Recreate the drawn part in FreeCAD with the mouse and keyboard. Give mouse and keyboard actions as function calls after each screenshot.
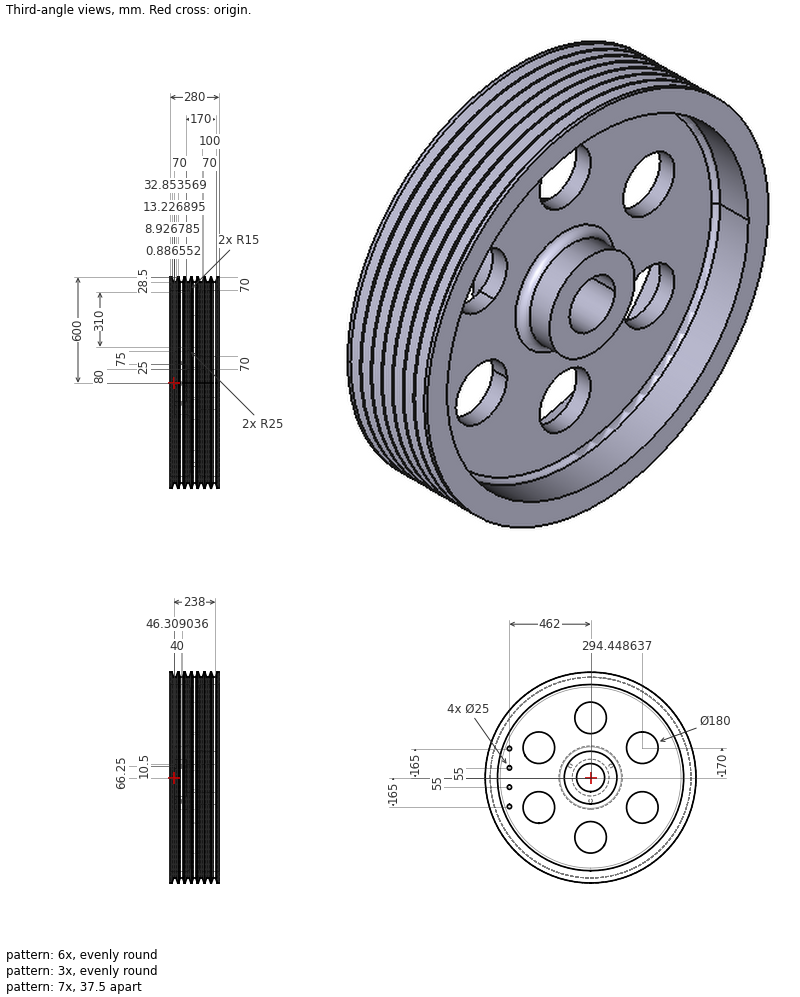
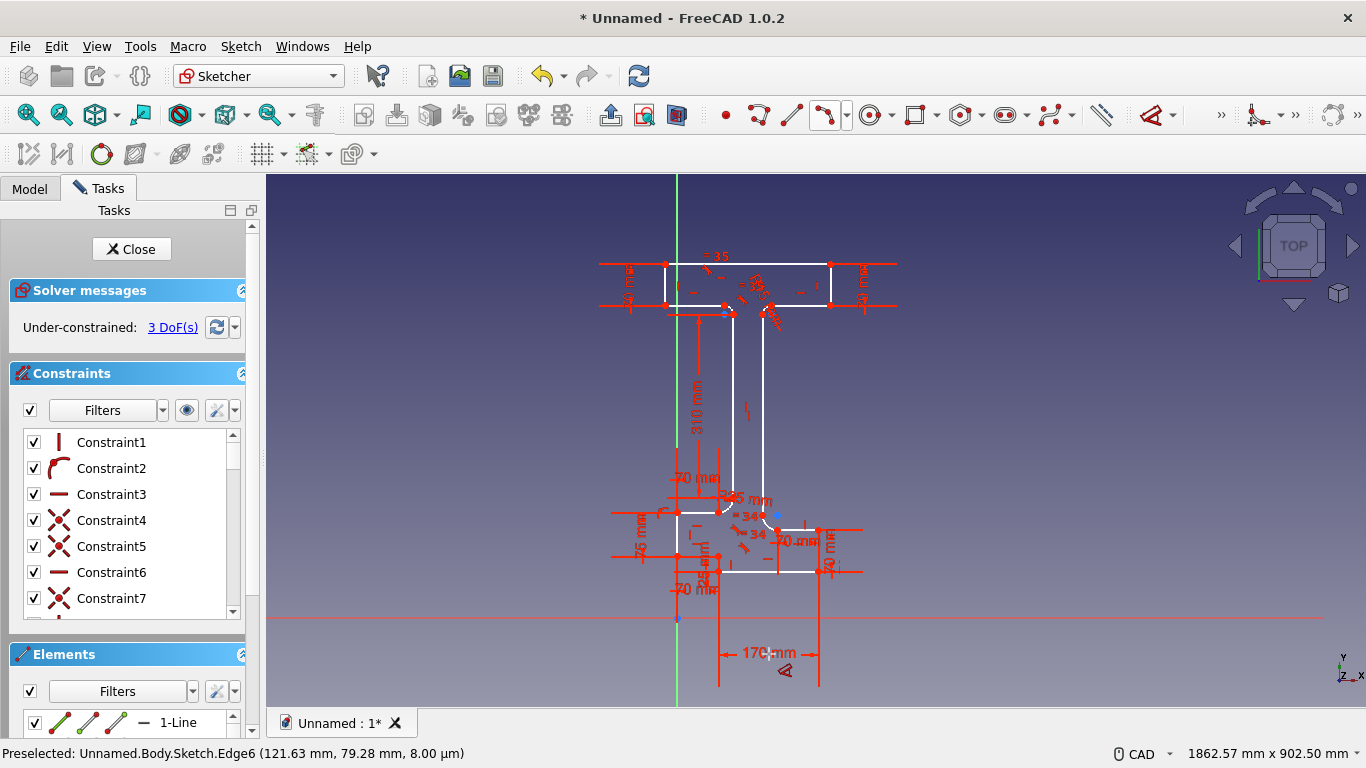
click(789, 306)
click(801, 340)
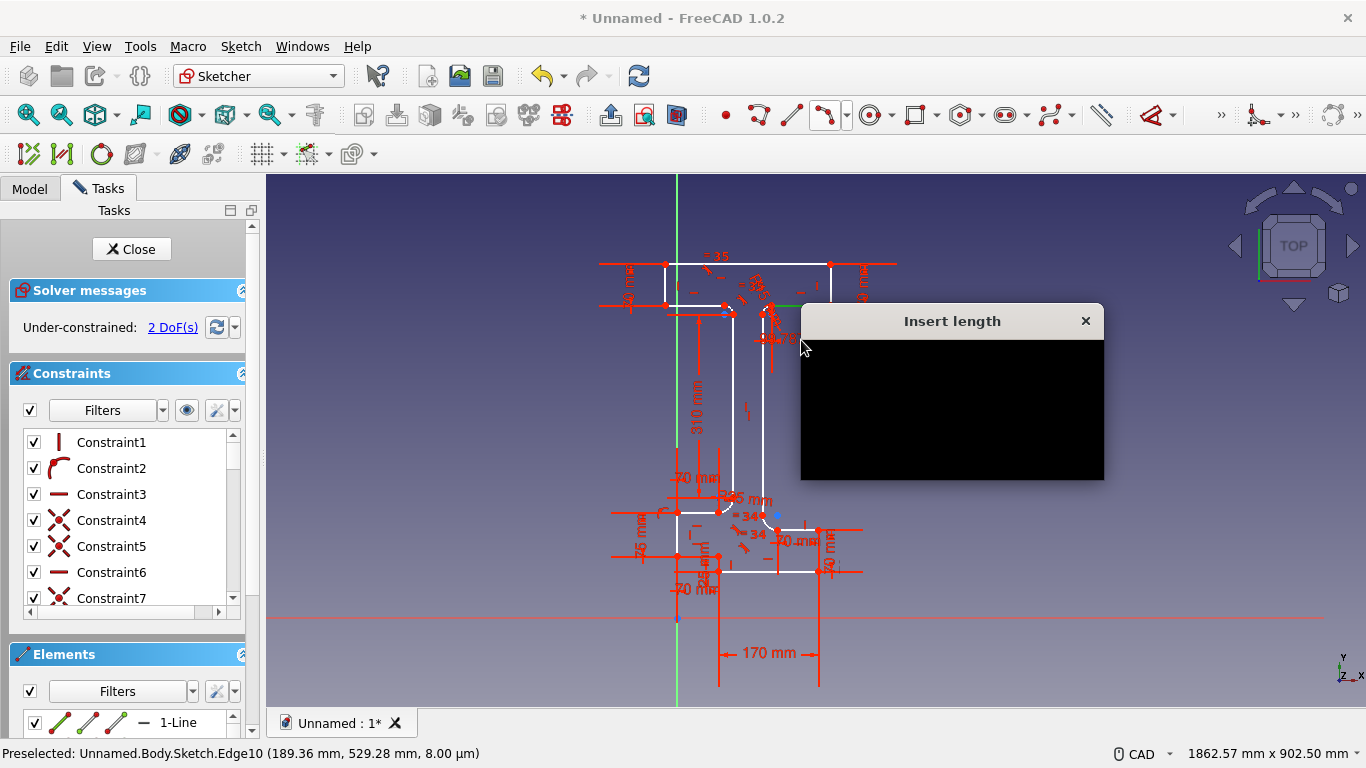
text(100)
key(Return)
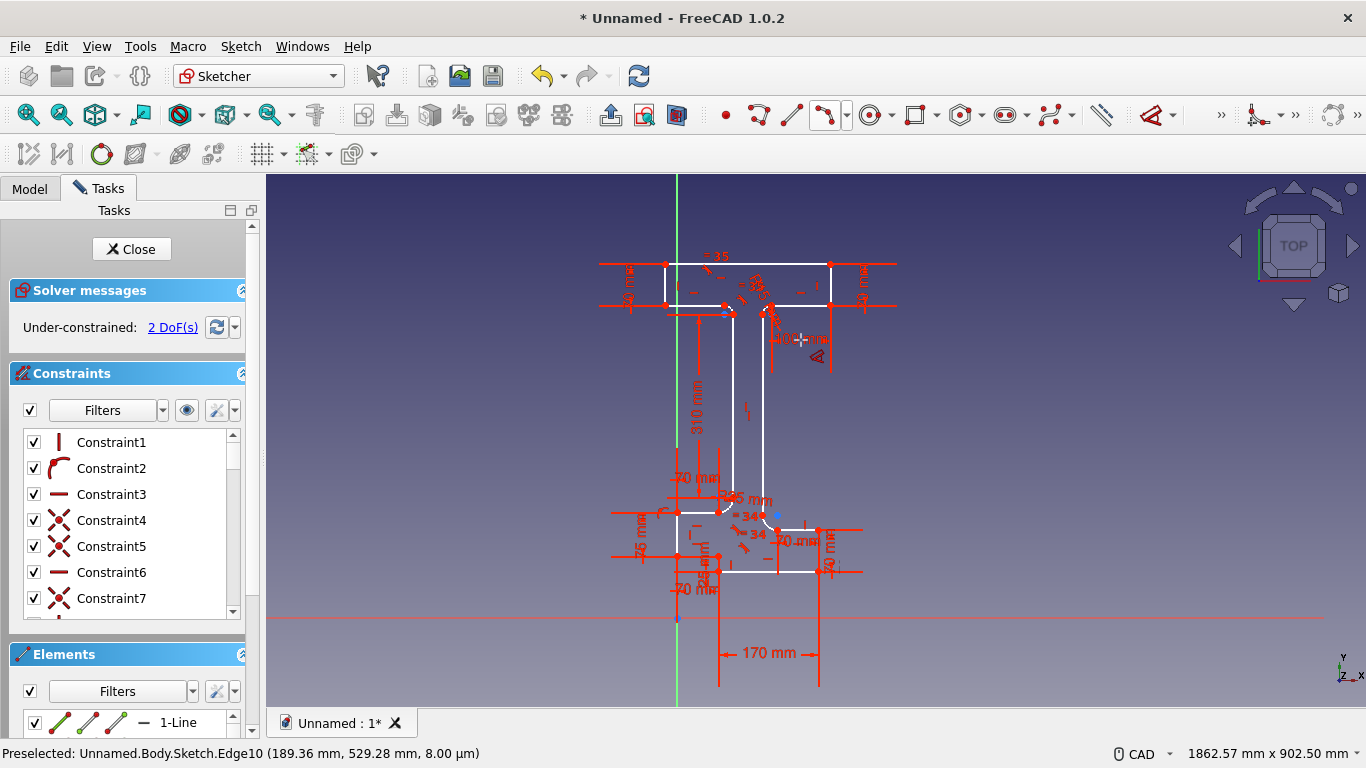
click(781, 264)
click(748, 230)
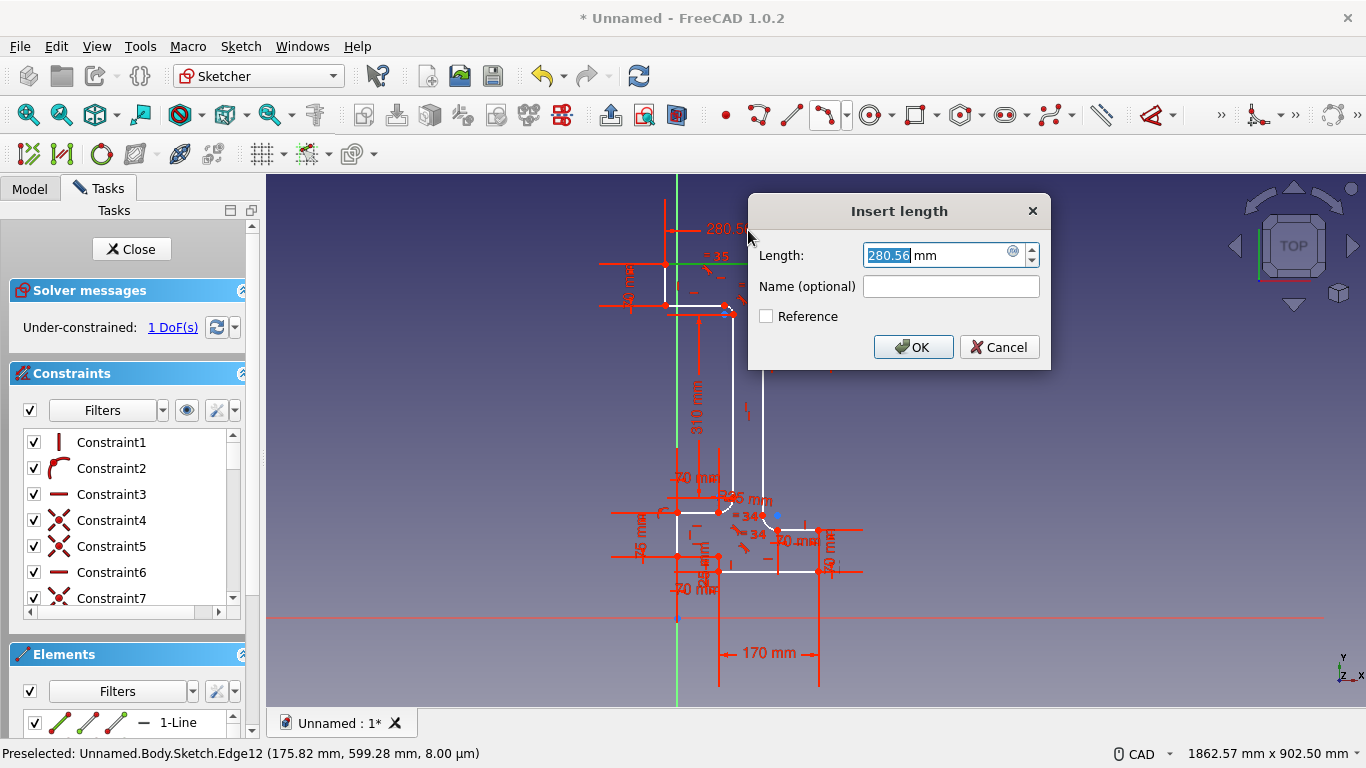
text(280)
key(Return)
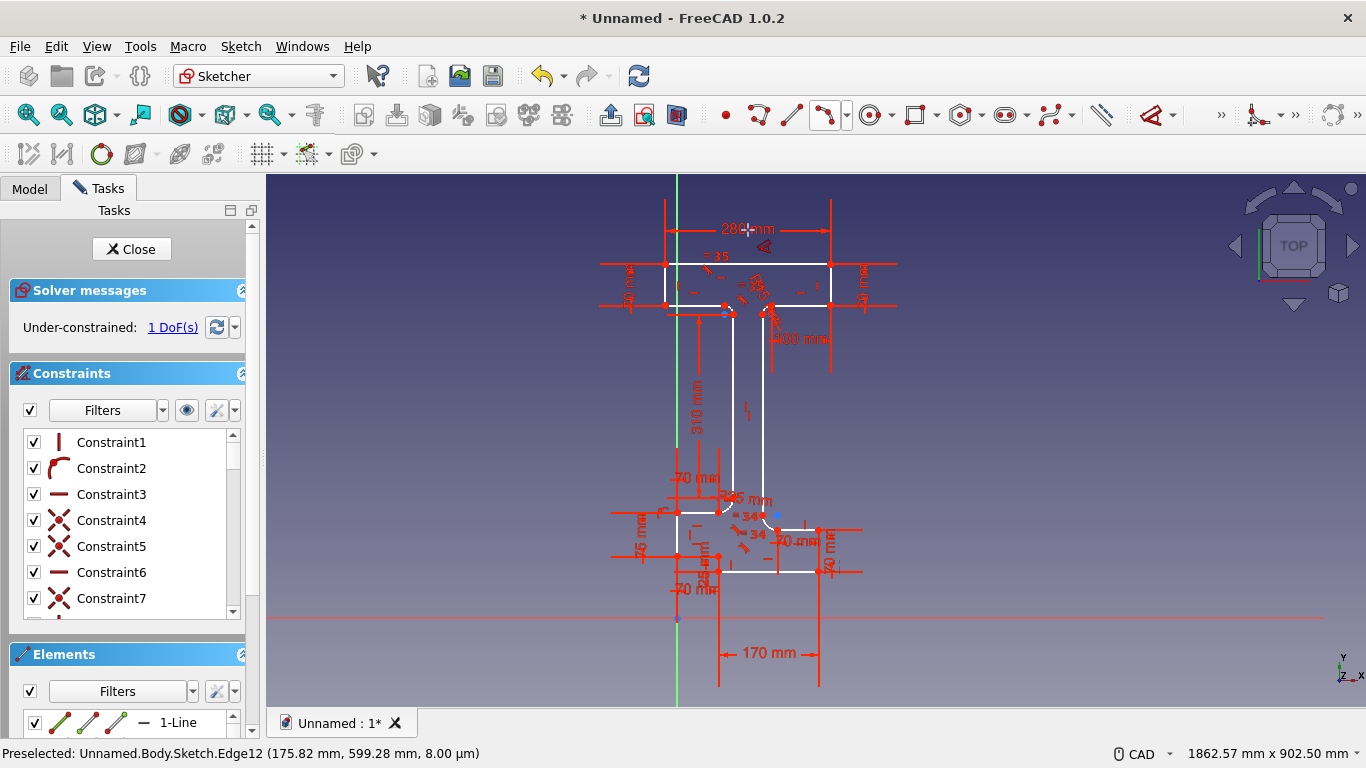
click(719, 572)
click(619, 595)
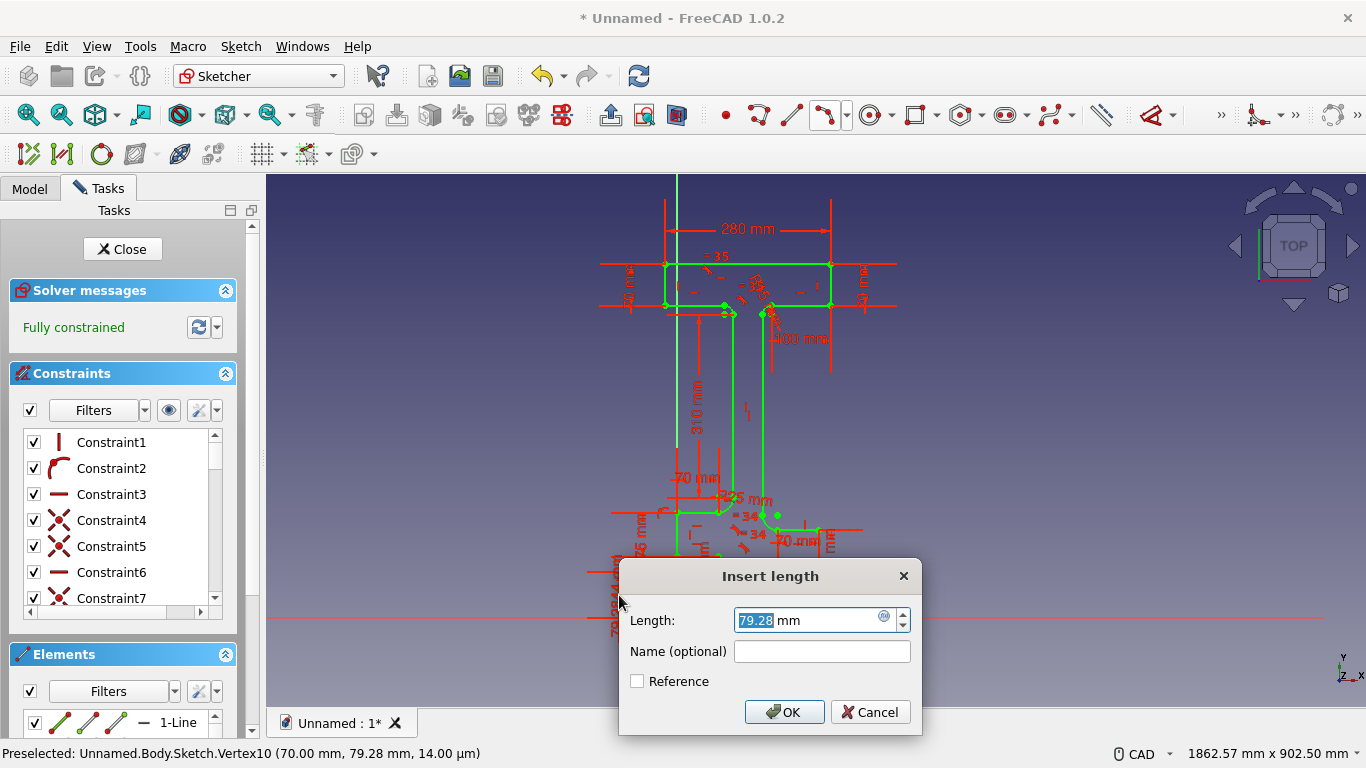
text(80)
key(Return)
key(Escape)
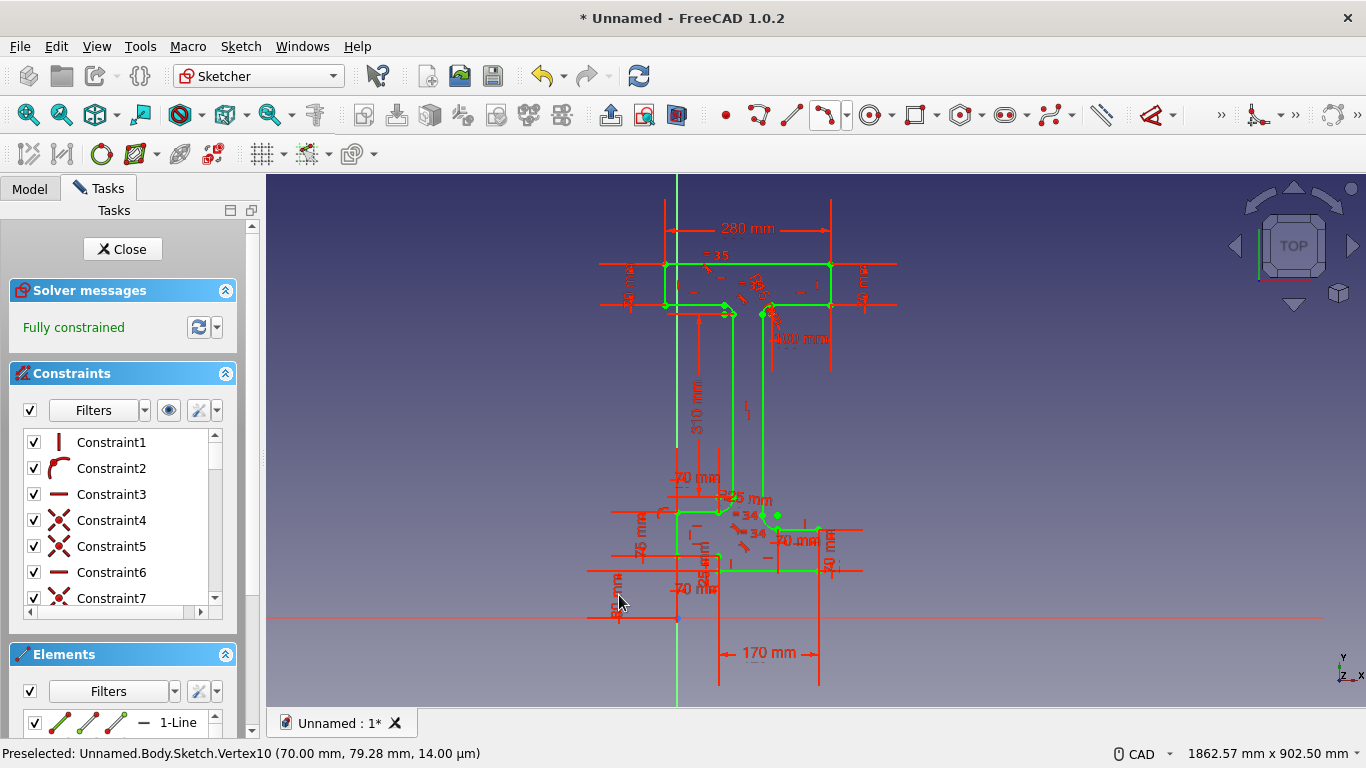
click(123, 249)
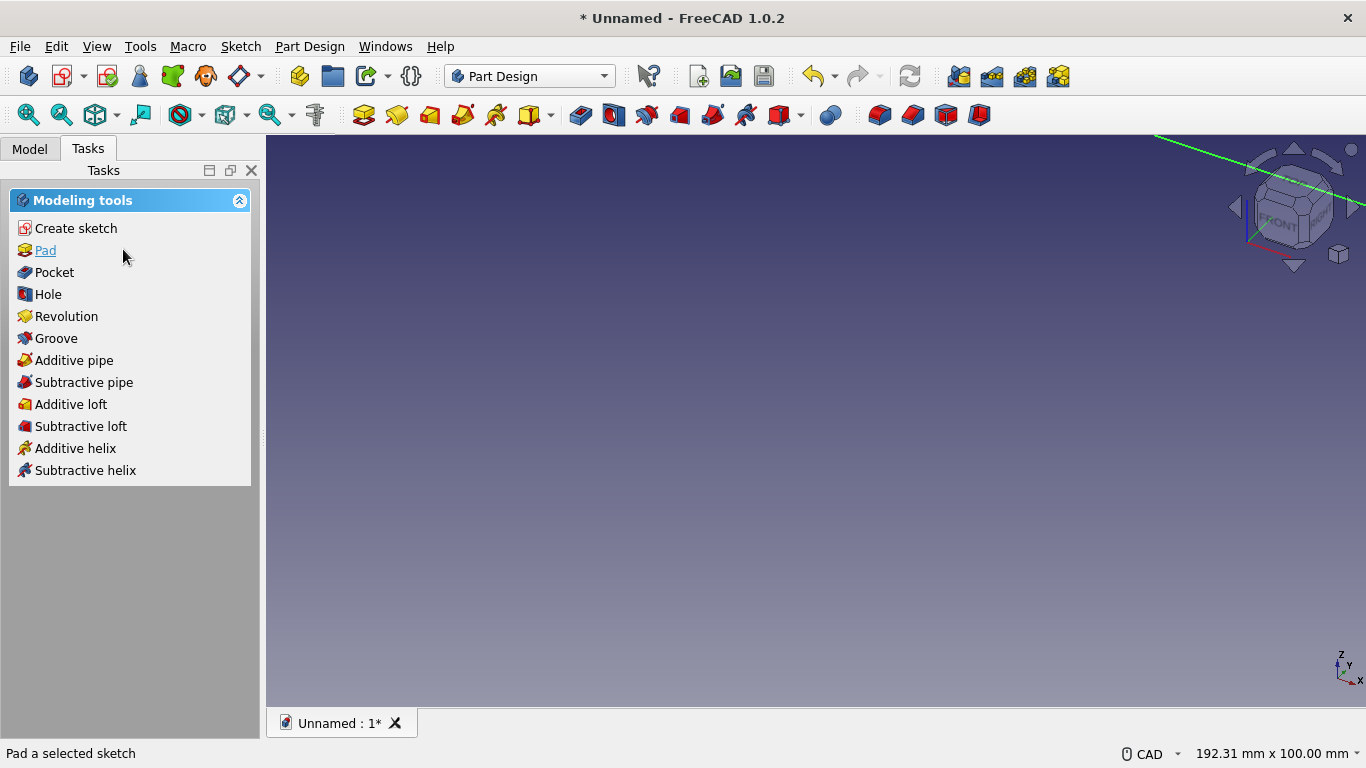
click(397, 116)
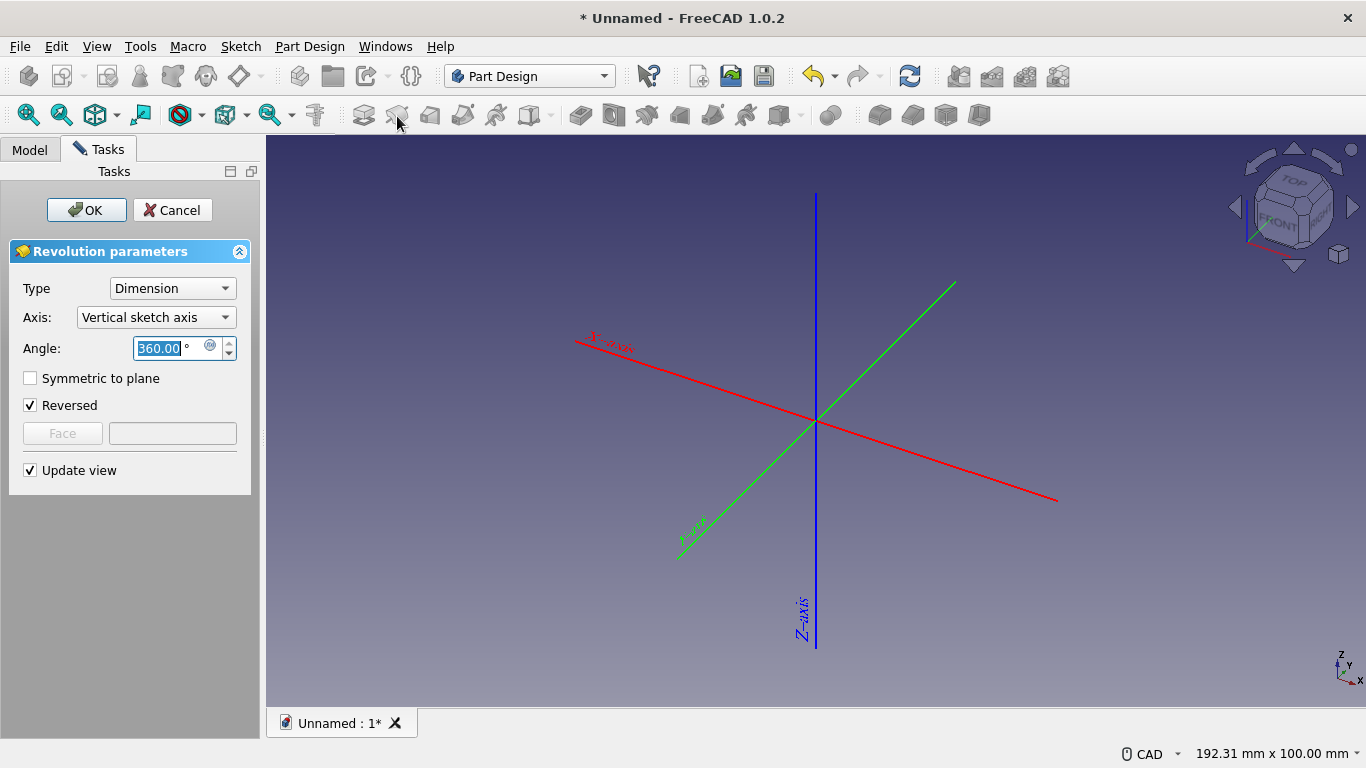
click(157, 318)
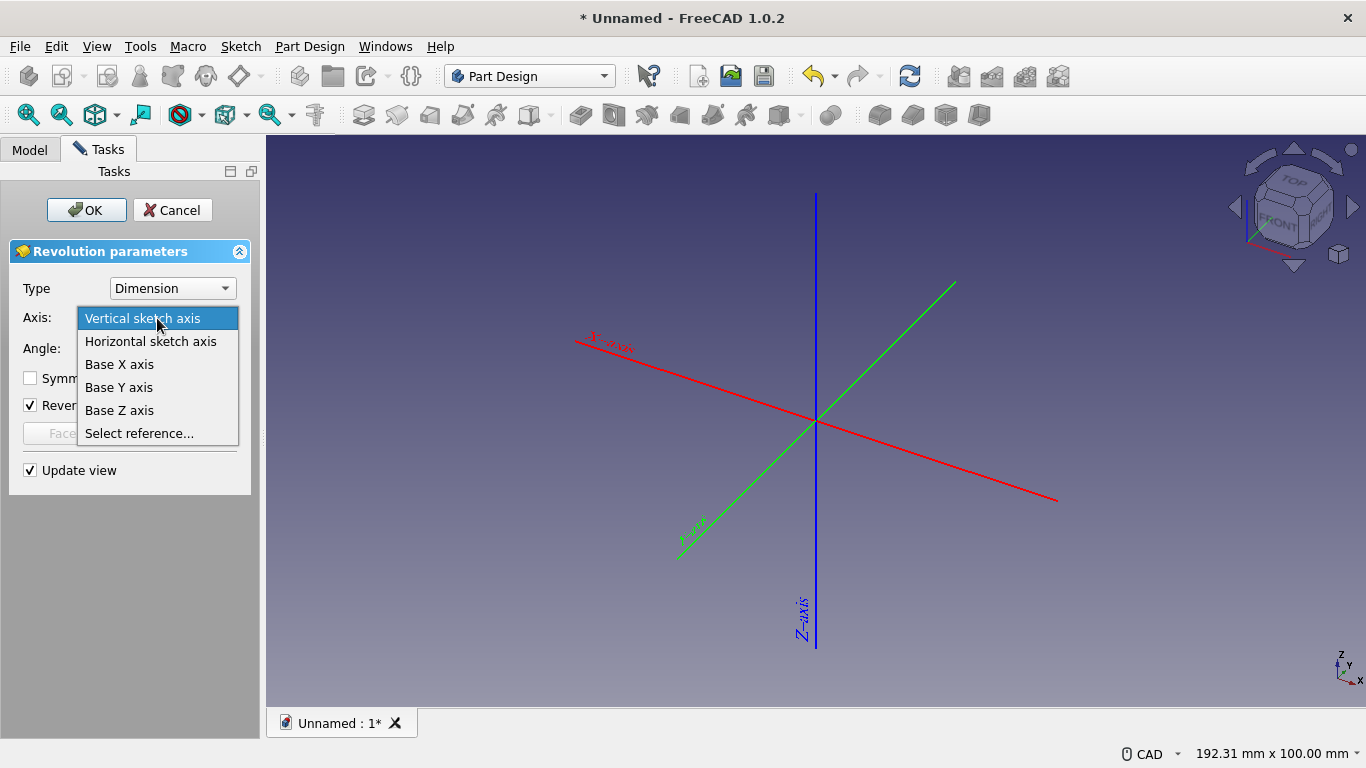
click(156, 342)